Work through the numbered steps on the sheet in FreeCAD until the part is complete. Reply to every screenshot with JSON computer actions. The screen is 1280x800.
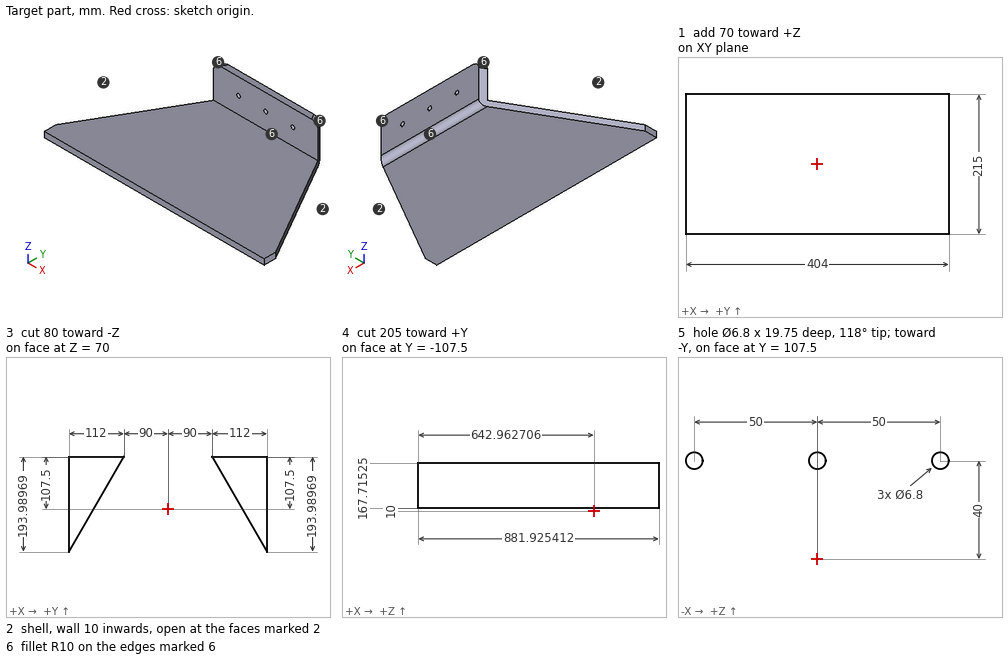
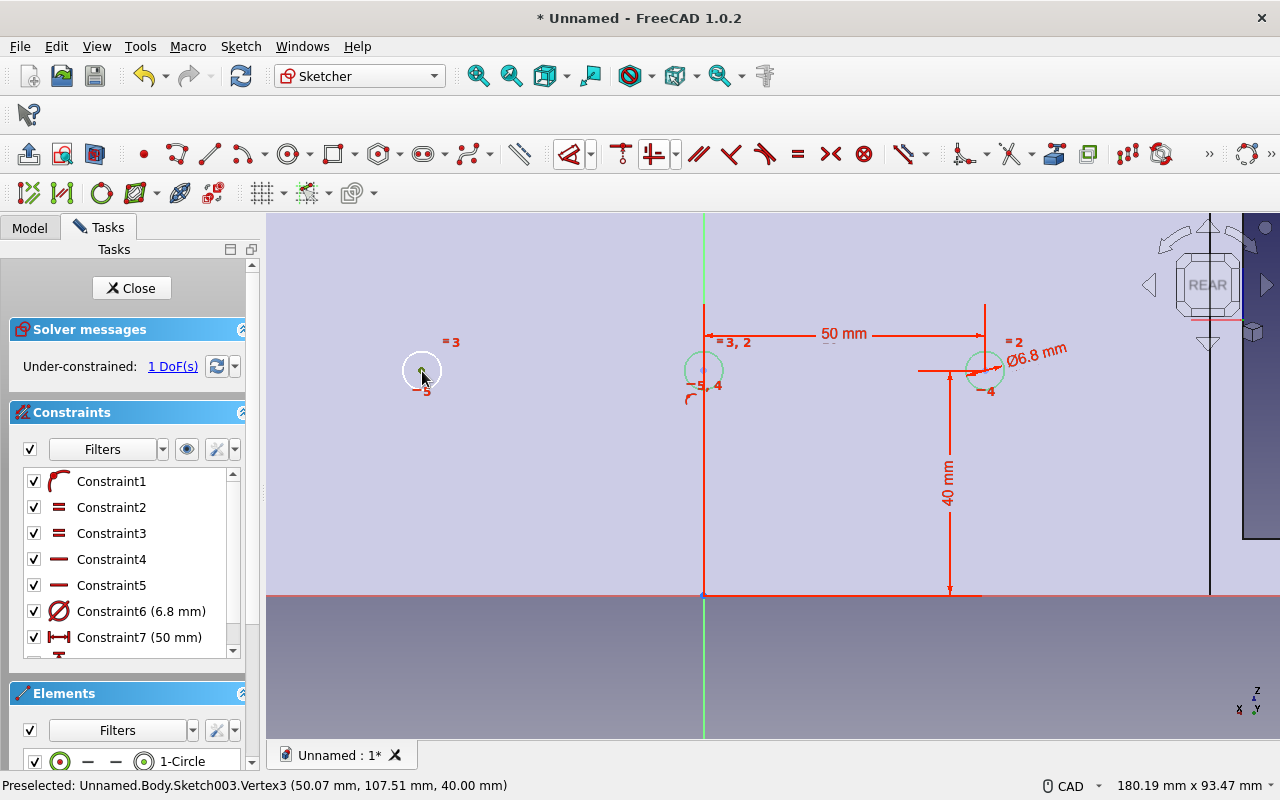
{"action": "key", "text": "l"}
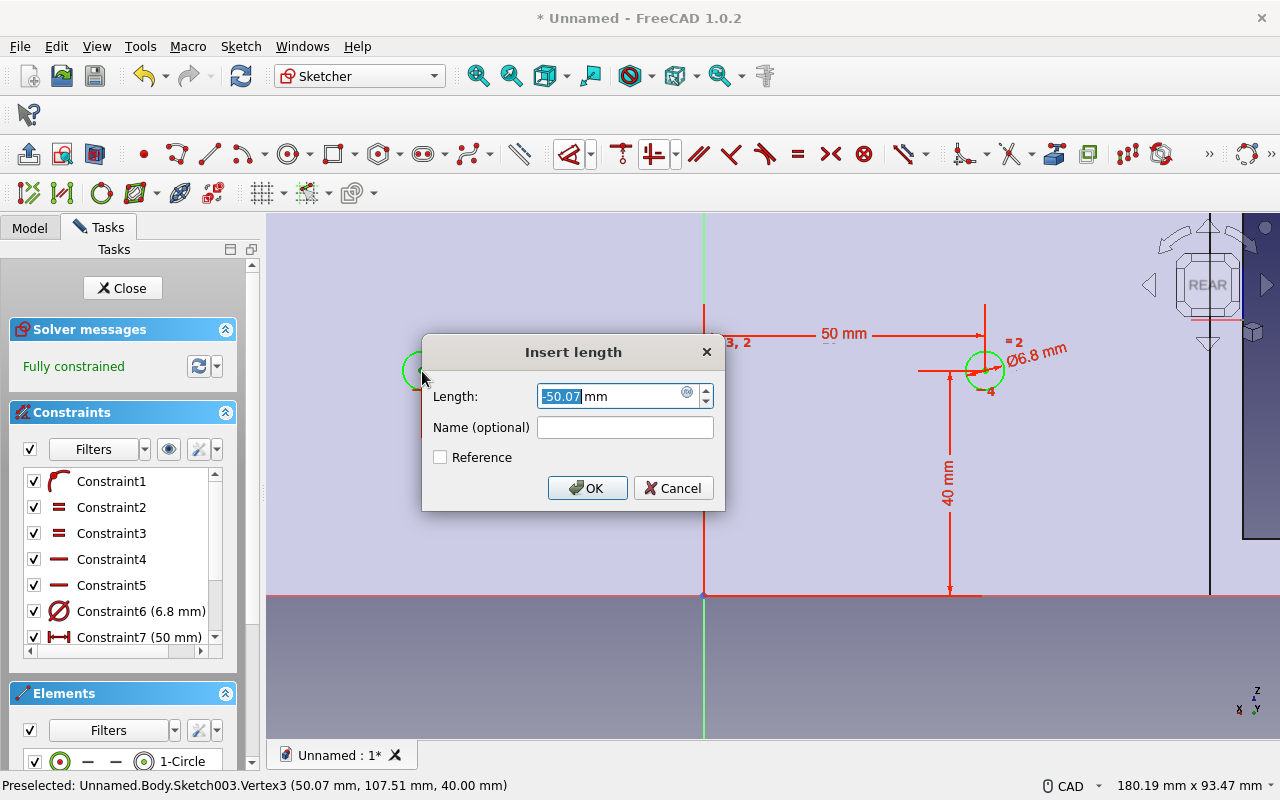
{"action": "type", "text": "-50"}
{"action": "key", "text": "Return"}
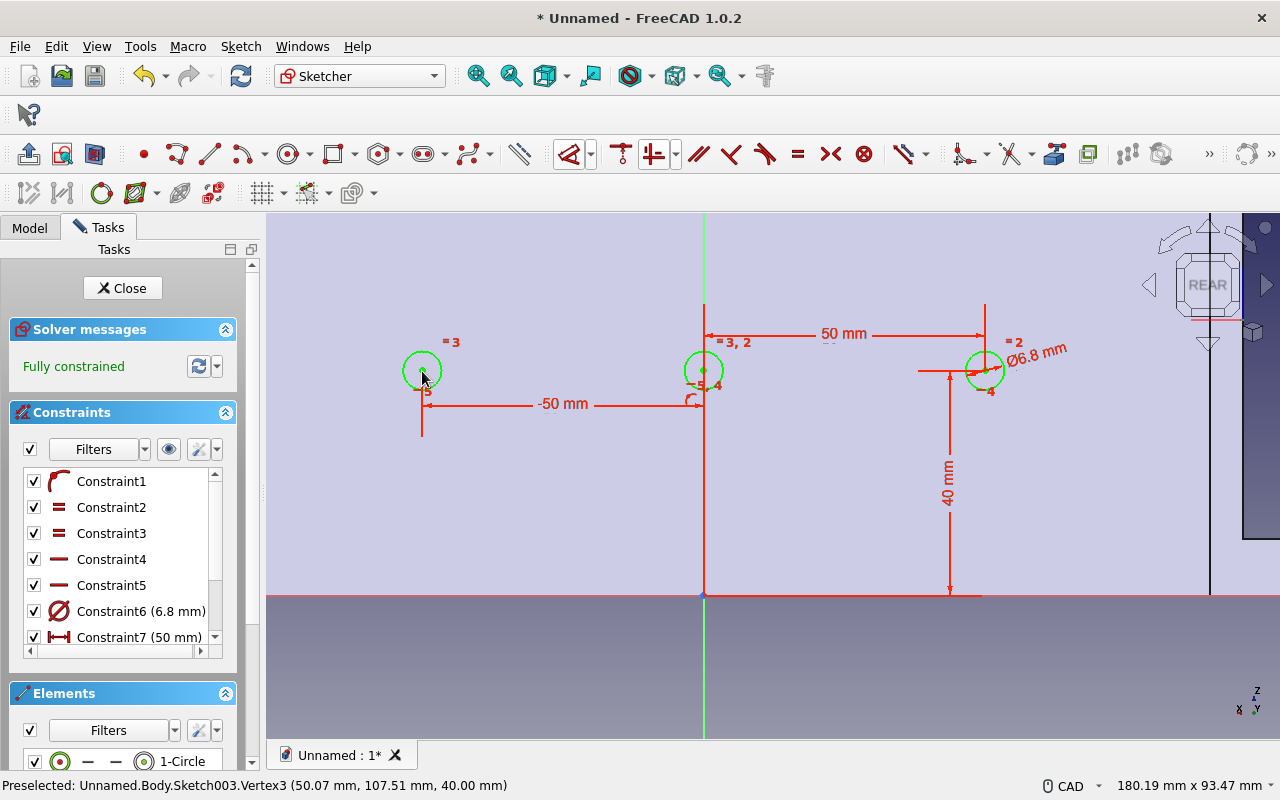
{"action": "left_click", "coordinate": [123, 288]}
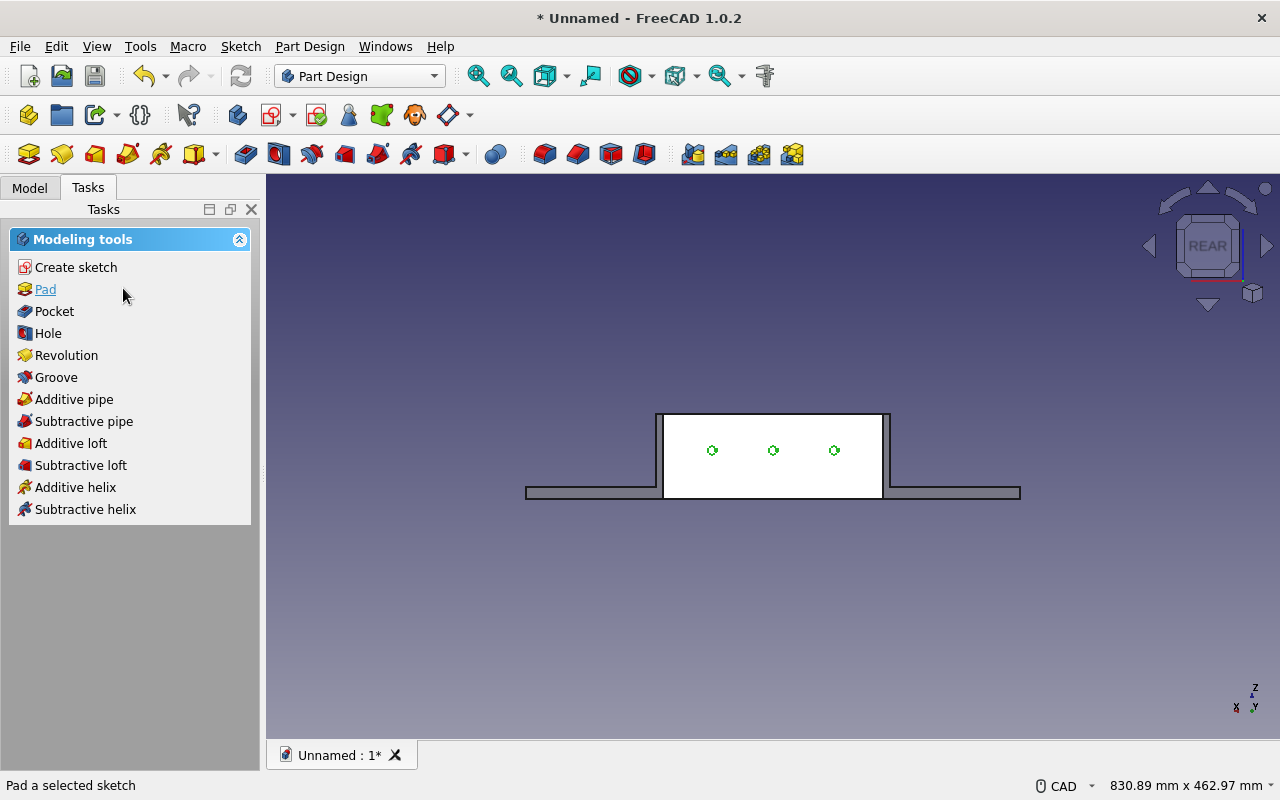
{"action": "left_click", "coordinate": [279, 154]}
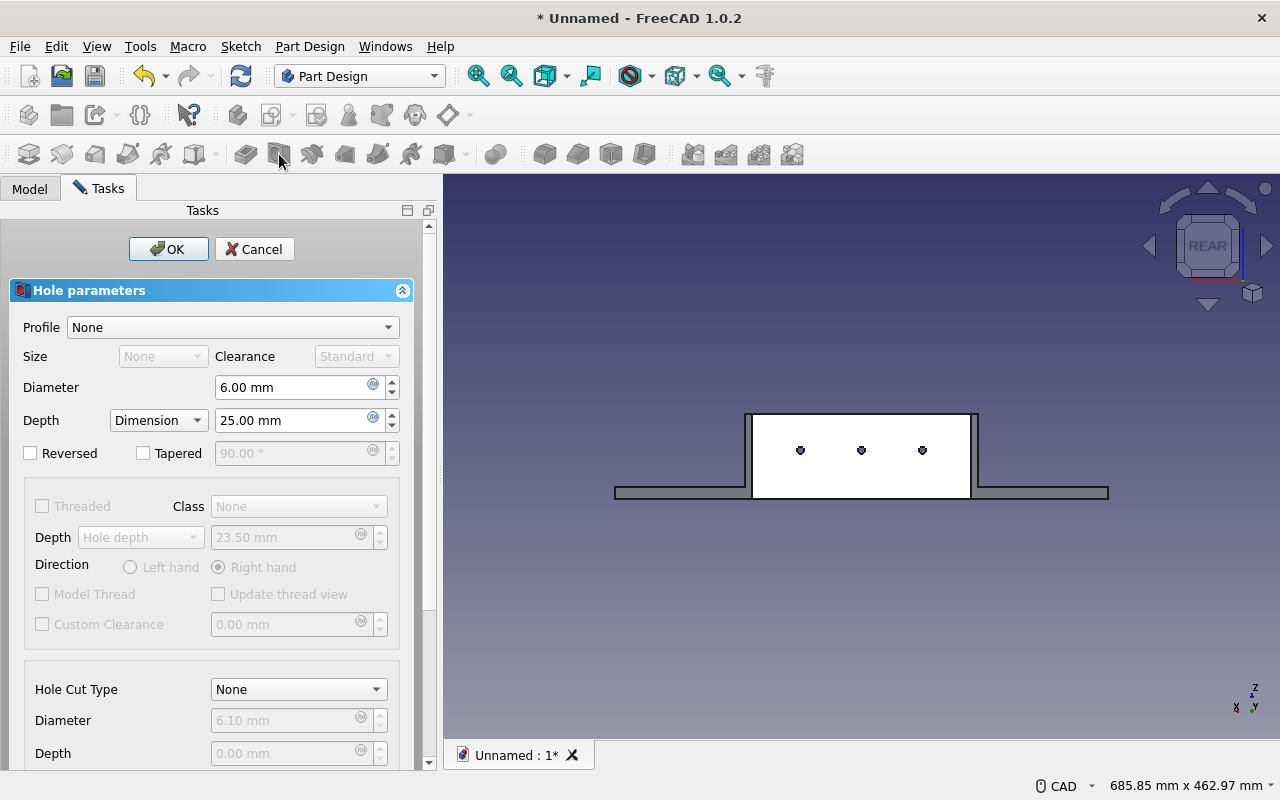
{"action": "triple_click", "coordinate": [300, 388]}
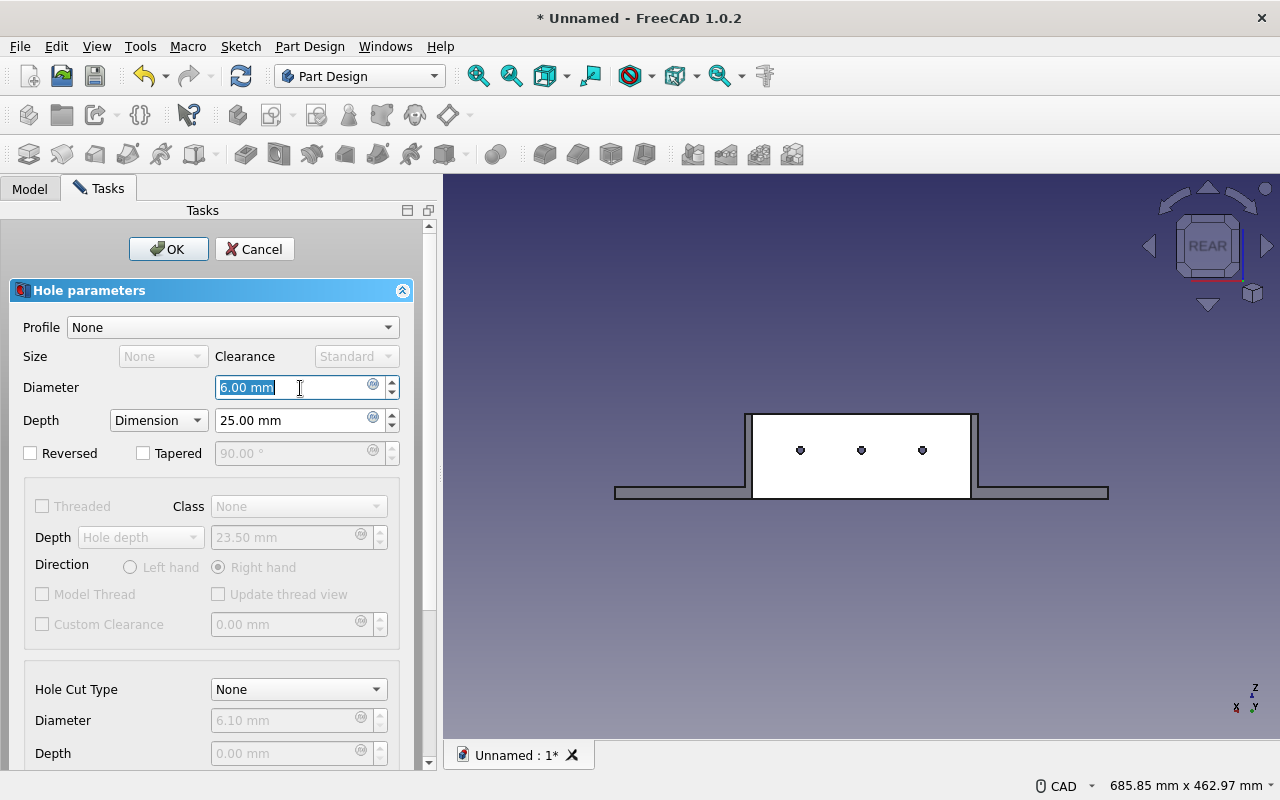
{"action": "type", "text": "6.8"}
{"action": "key", "text": "Tab"}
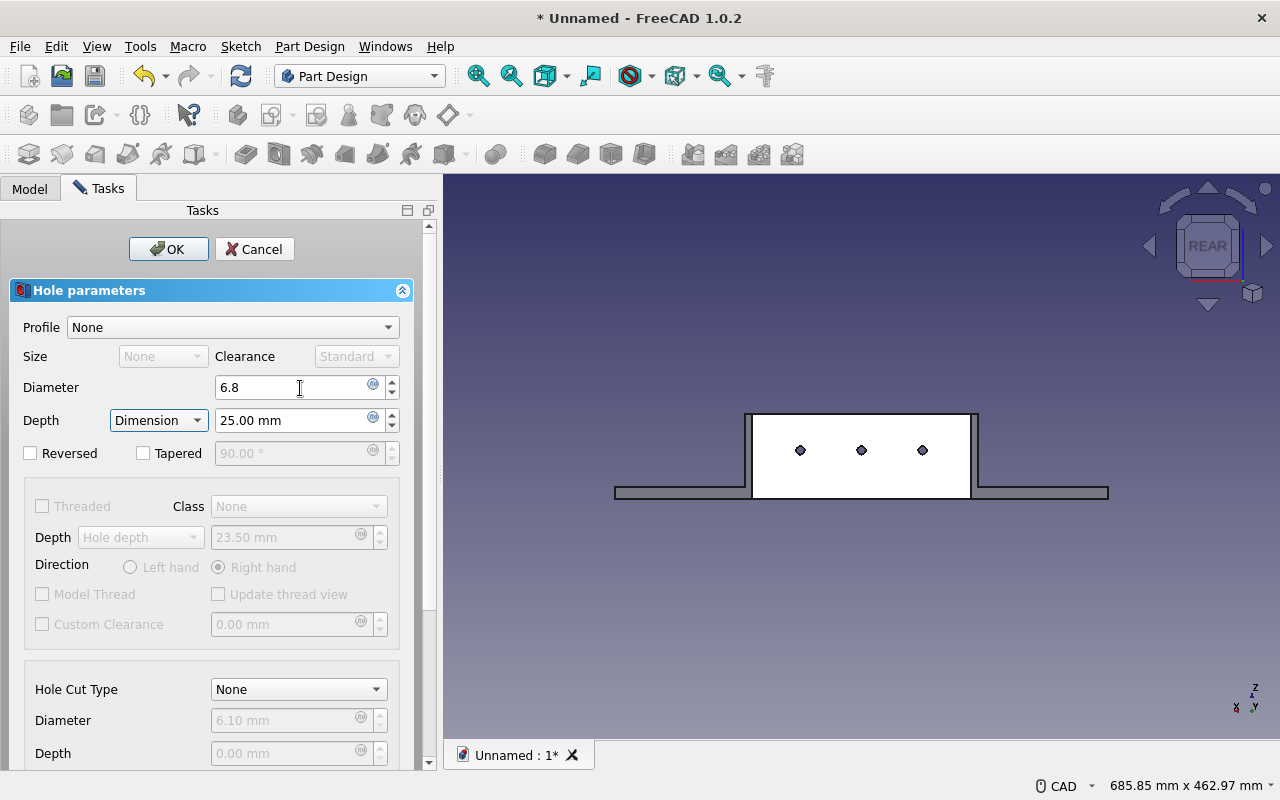
{"action": "triple_click", "coordinate": [300, 420]}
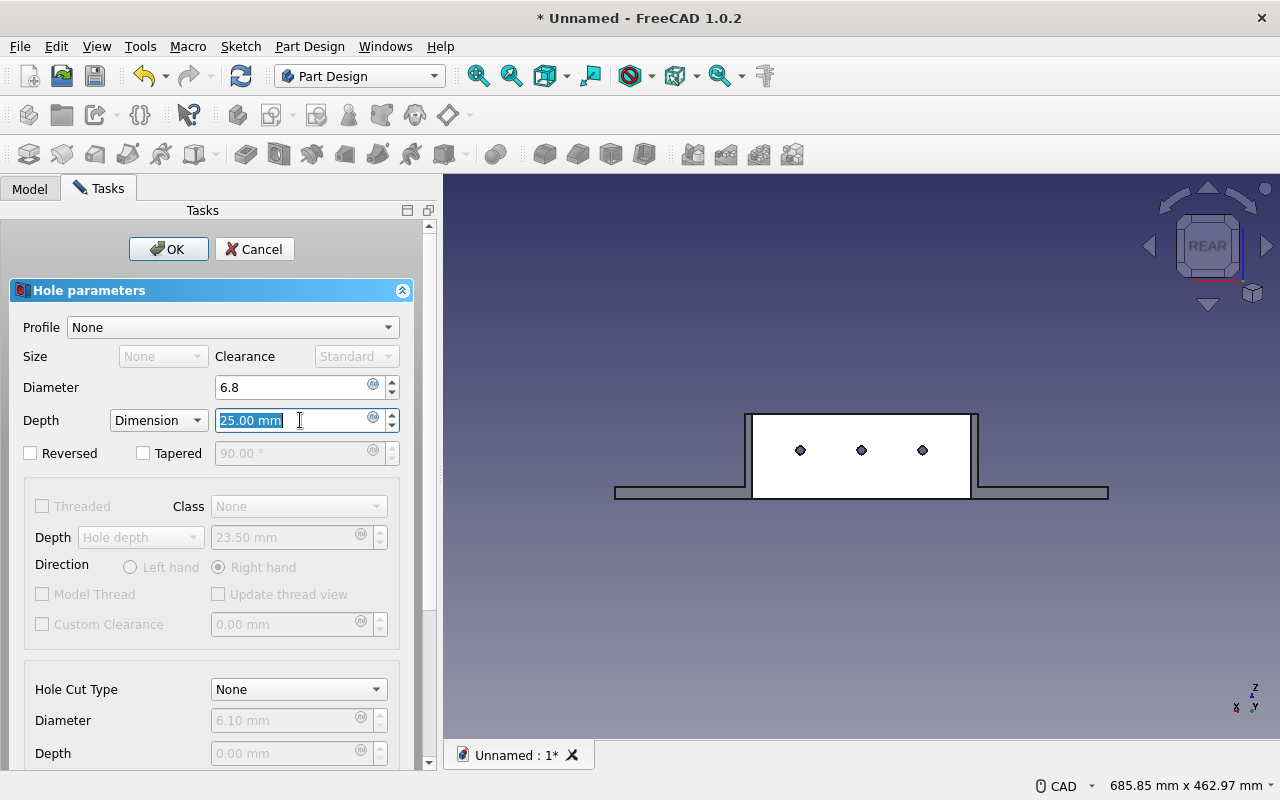
{"action": "type", "text": "19.75"}
{"action": "key", "text": "Tab"}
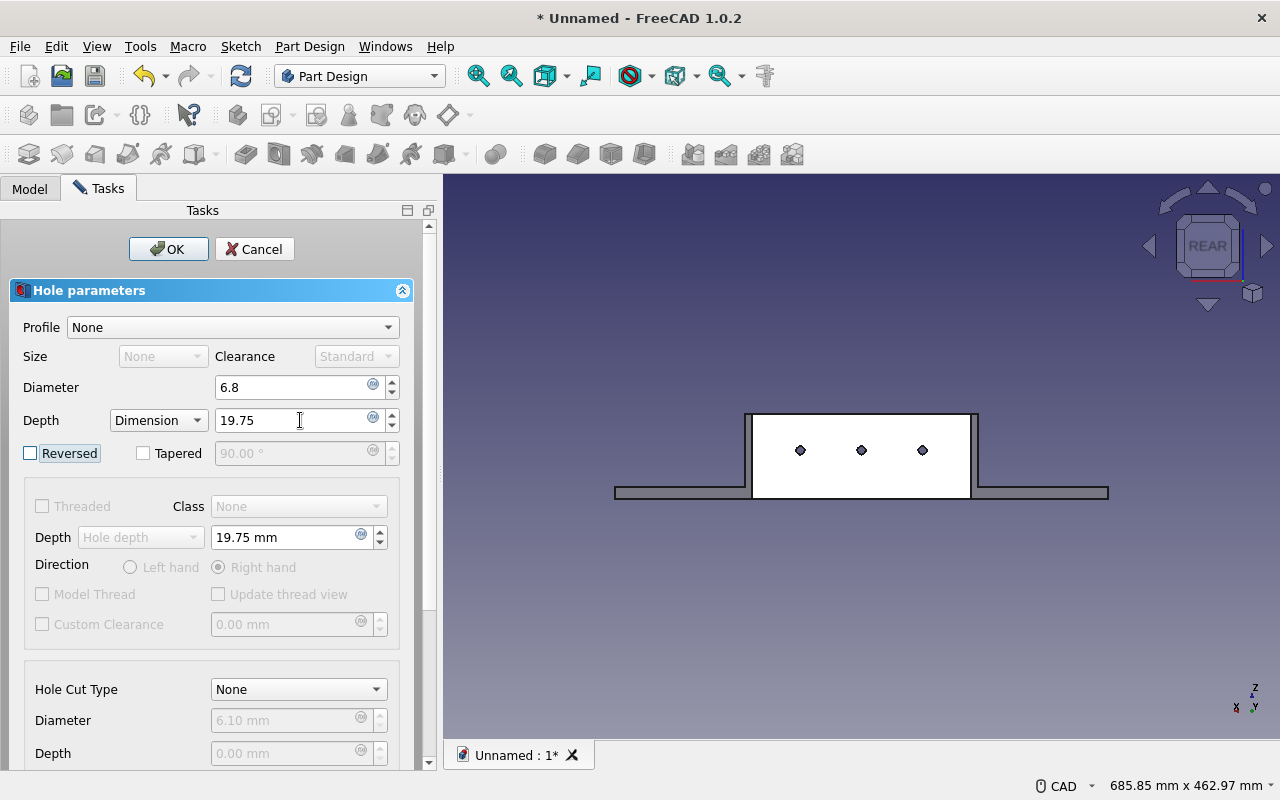
{"action": "left_click", "coordinate": [169, 249]}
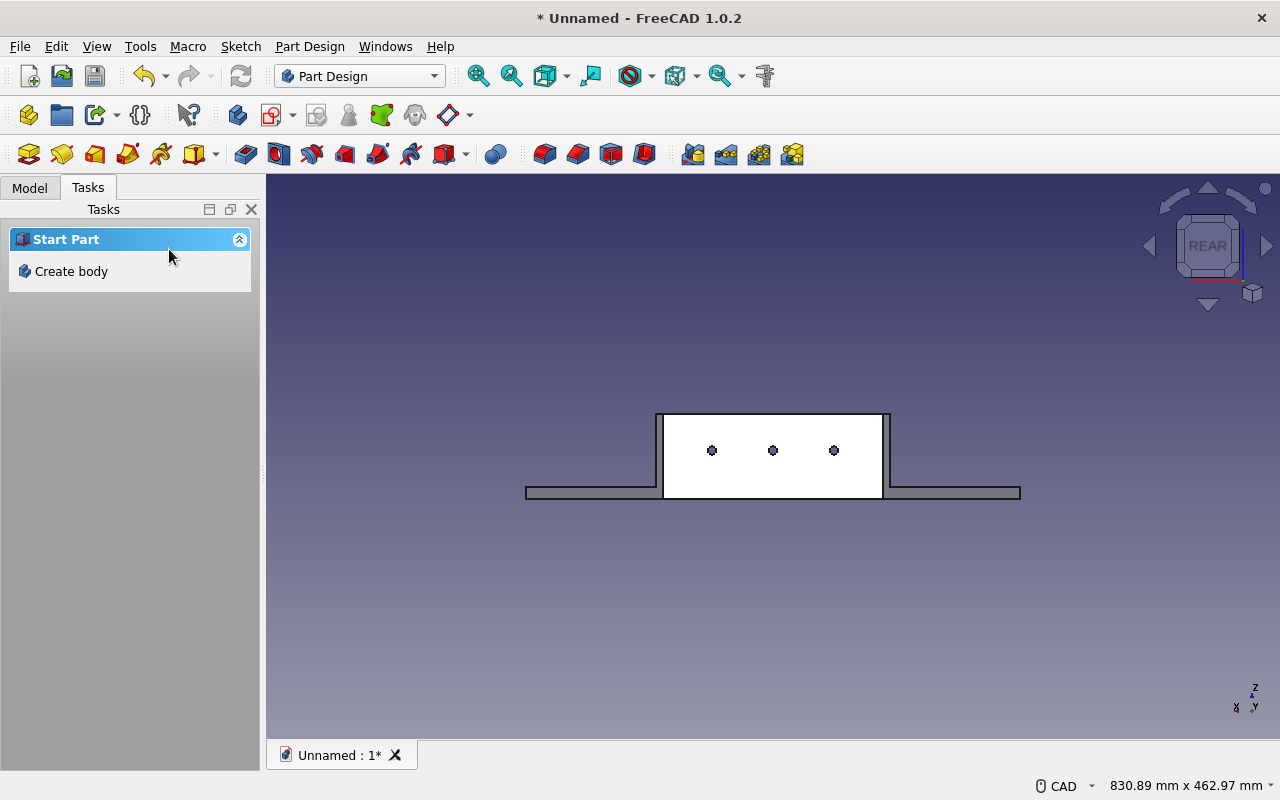
{"action": "left_click", "coordinate": [773, 498]}